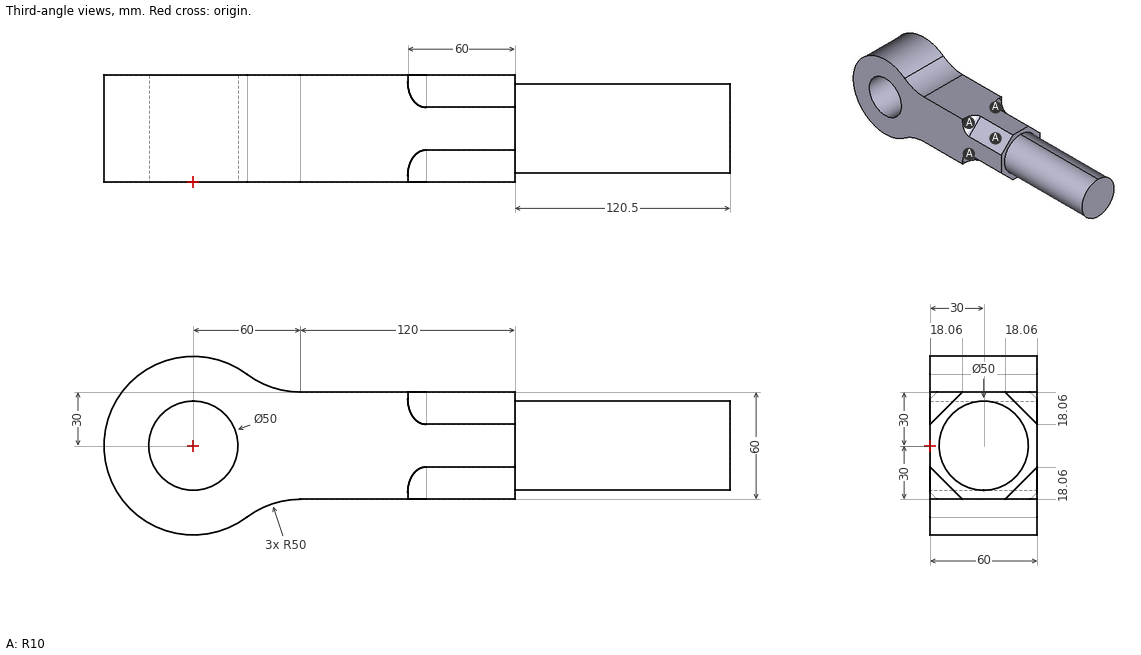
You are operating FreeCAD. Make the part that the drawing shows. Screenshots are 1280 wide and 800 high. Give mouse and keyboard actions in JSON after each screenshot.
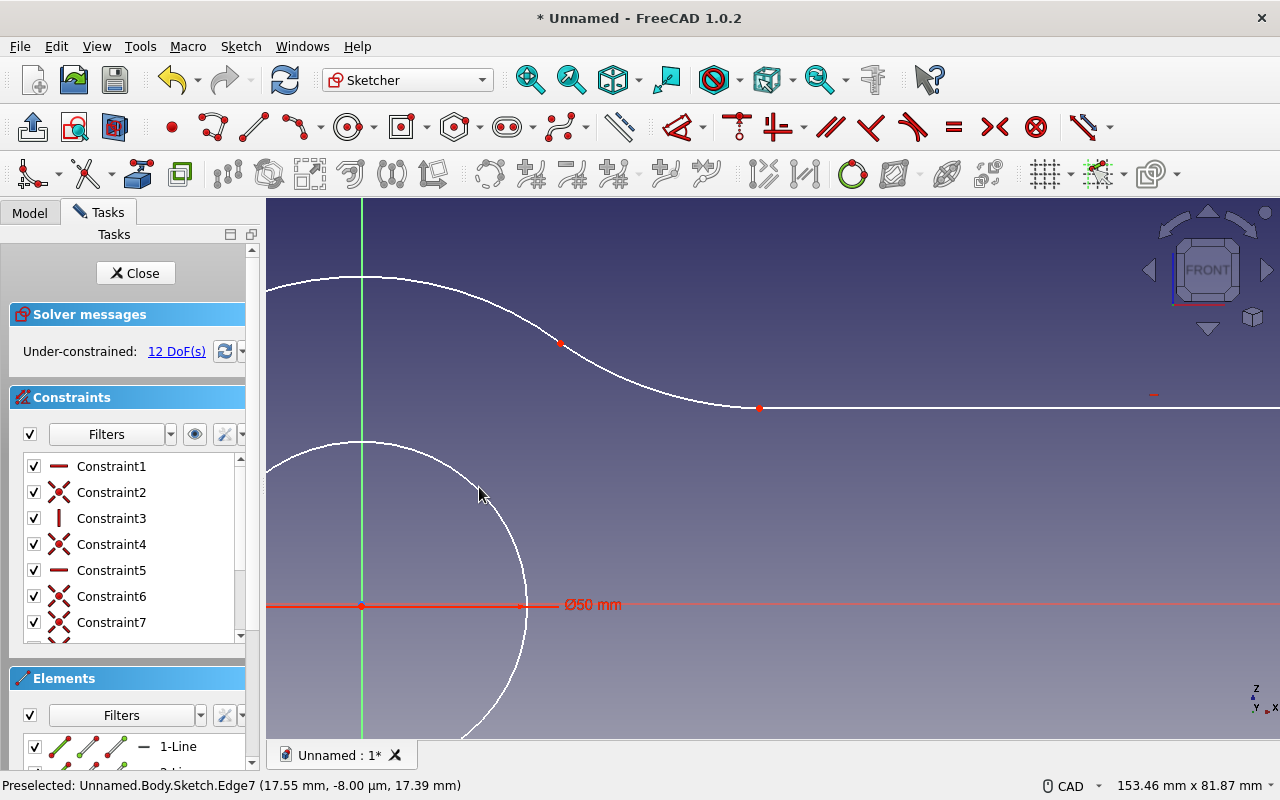
{"action": "scroll", "coordinate": [654, 389], "scroll_direction": "down", "scroll_amount": 5}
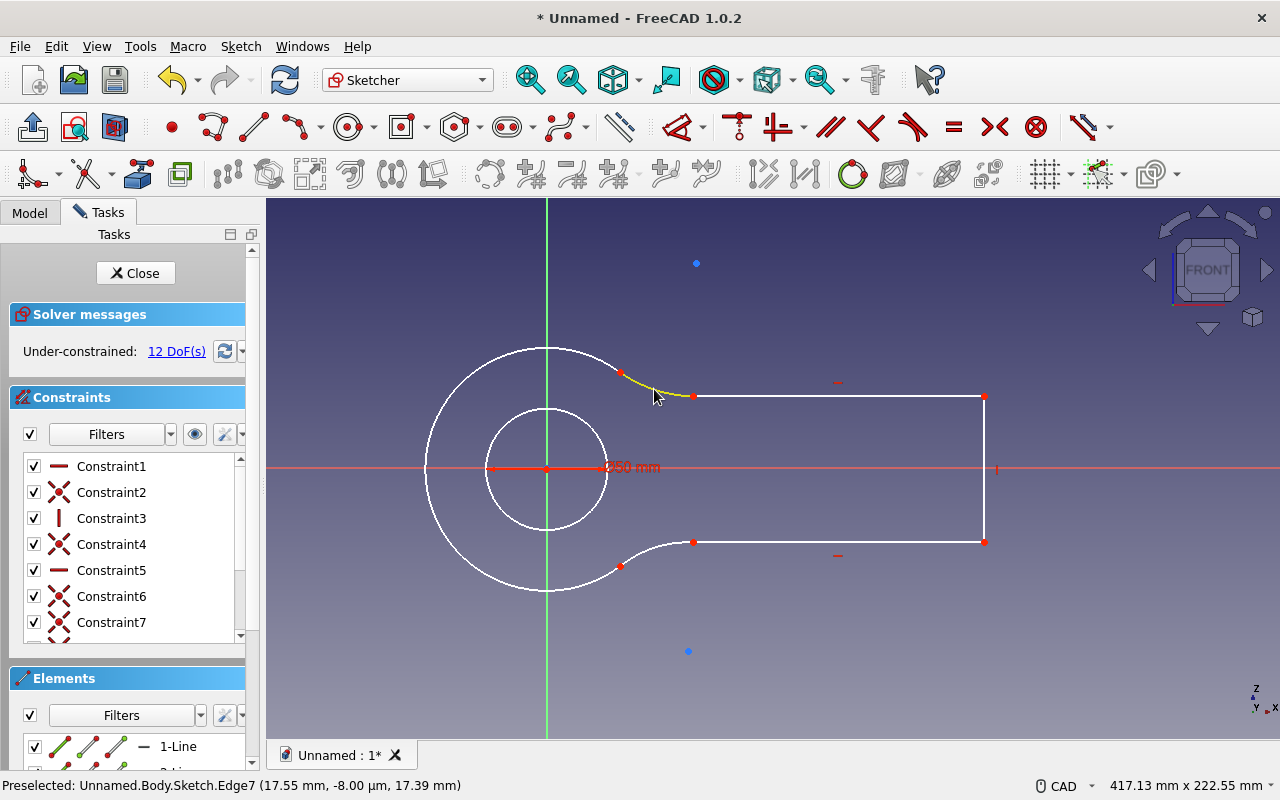
{"action": "left_click", "coordinate": [670, 544]}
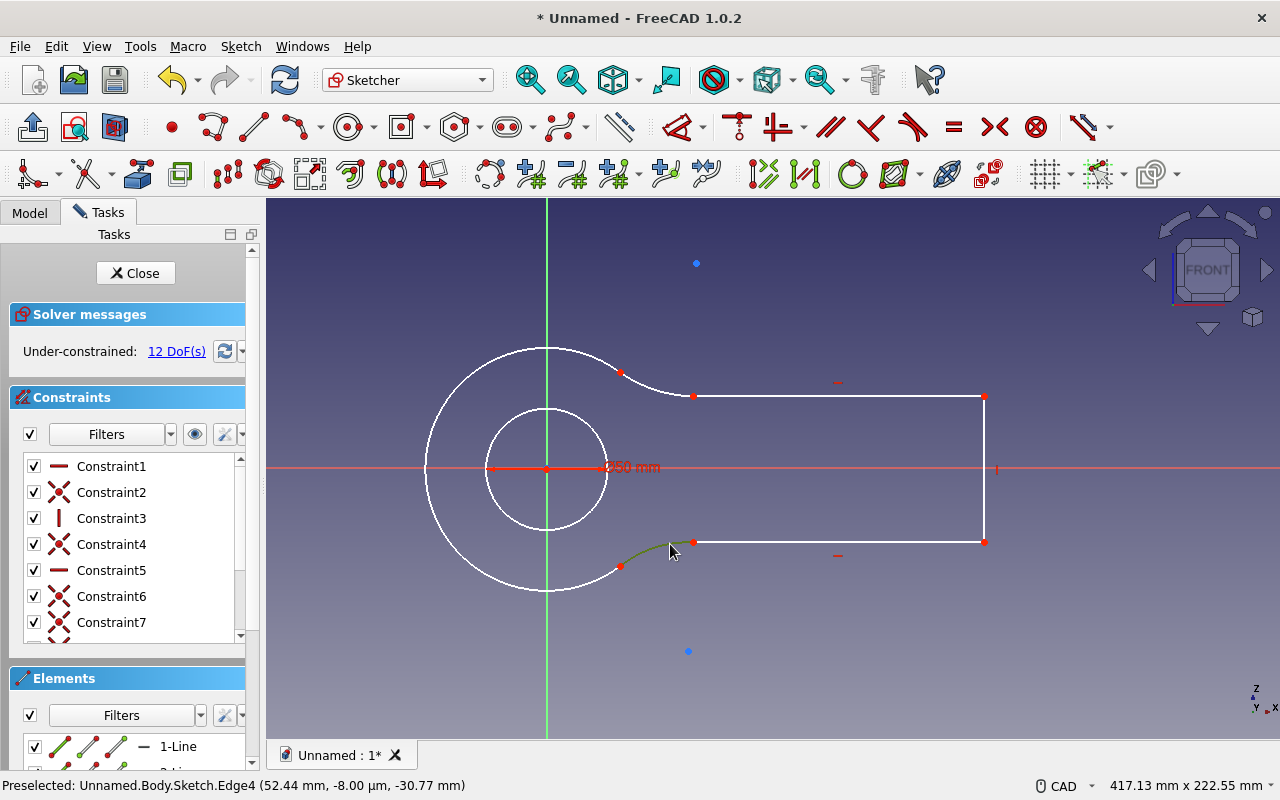
{"action": "left_click", "coordinate": [470, 375]}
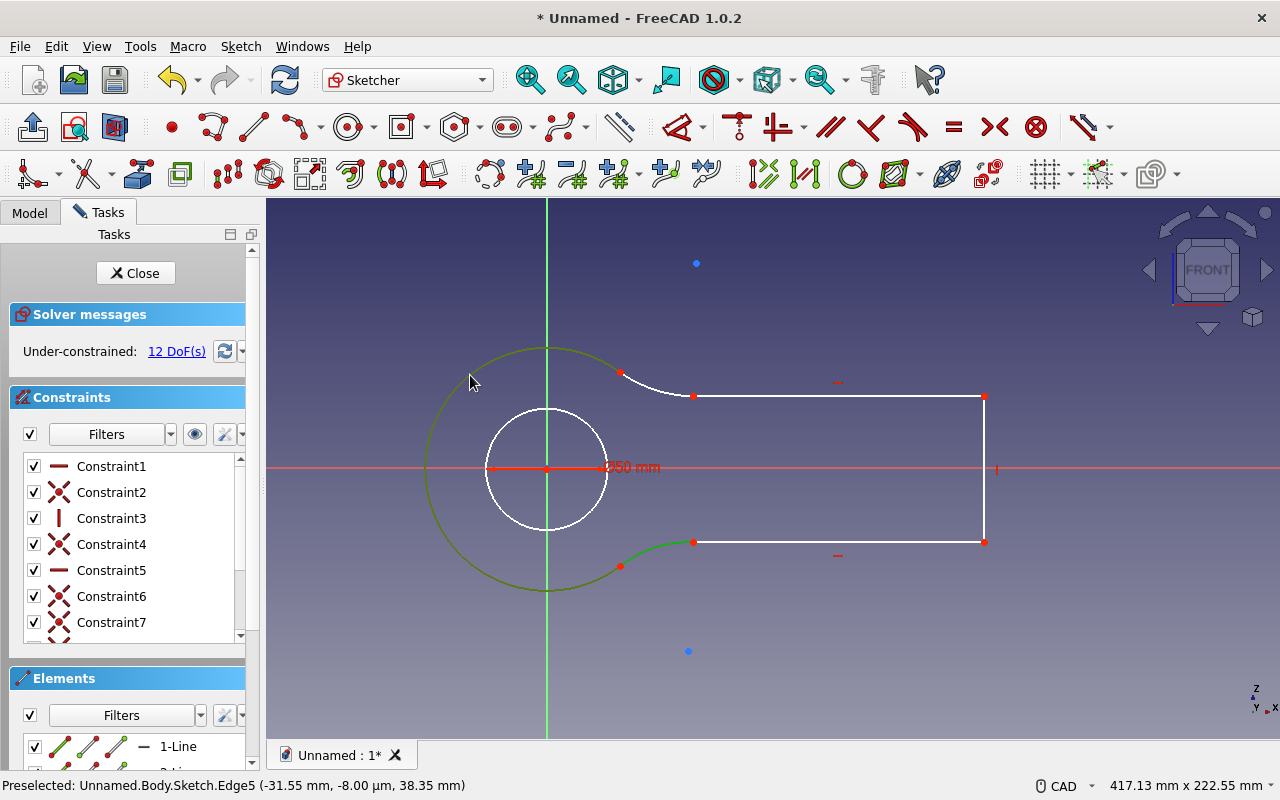
{"action": "key", "text": "t"}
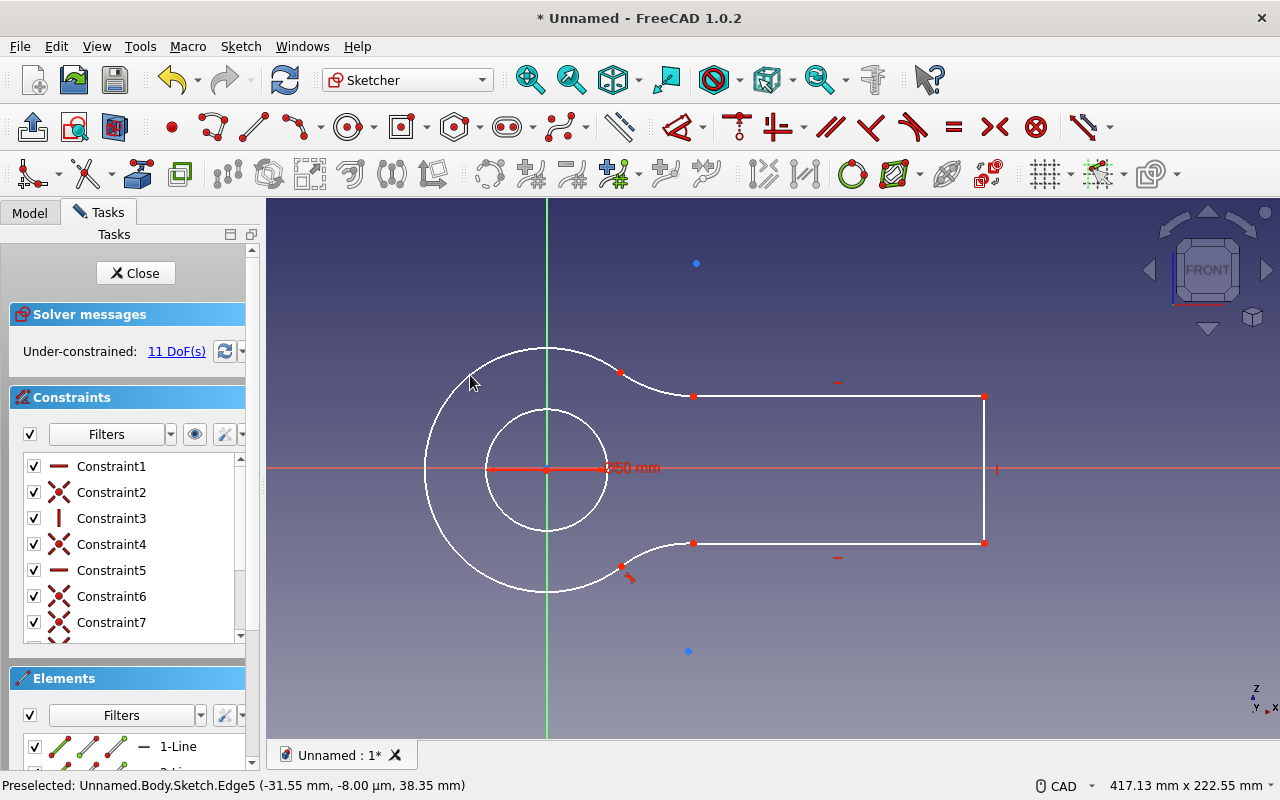
{"action": "left_click", "coordinate": [469, 376]}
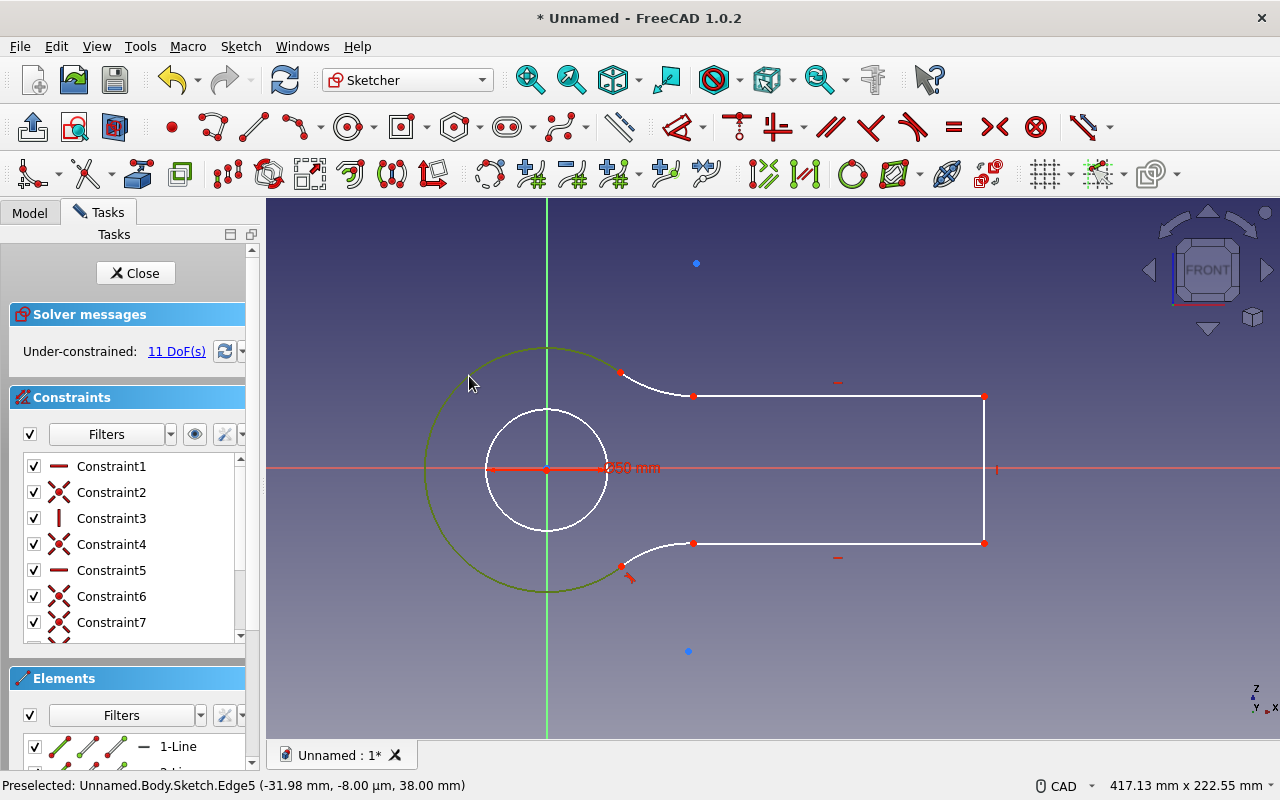
{"action": "left_click", "coordinate": [640, 384]}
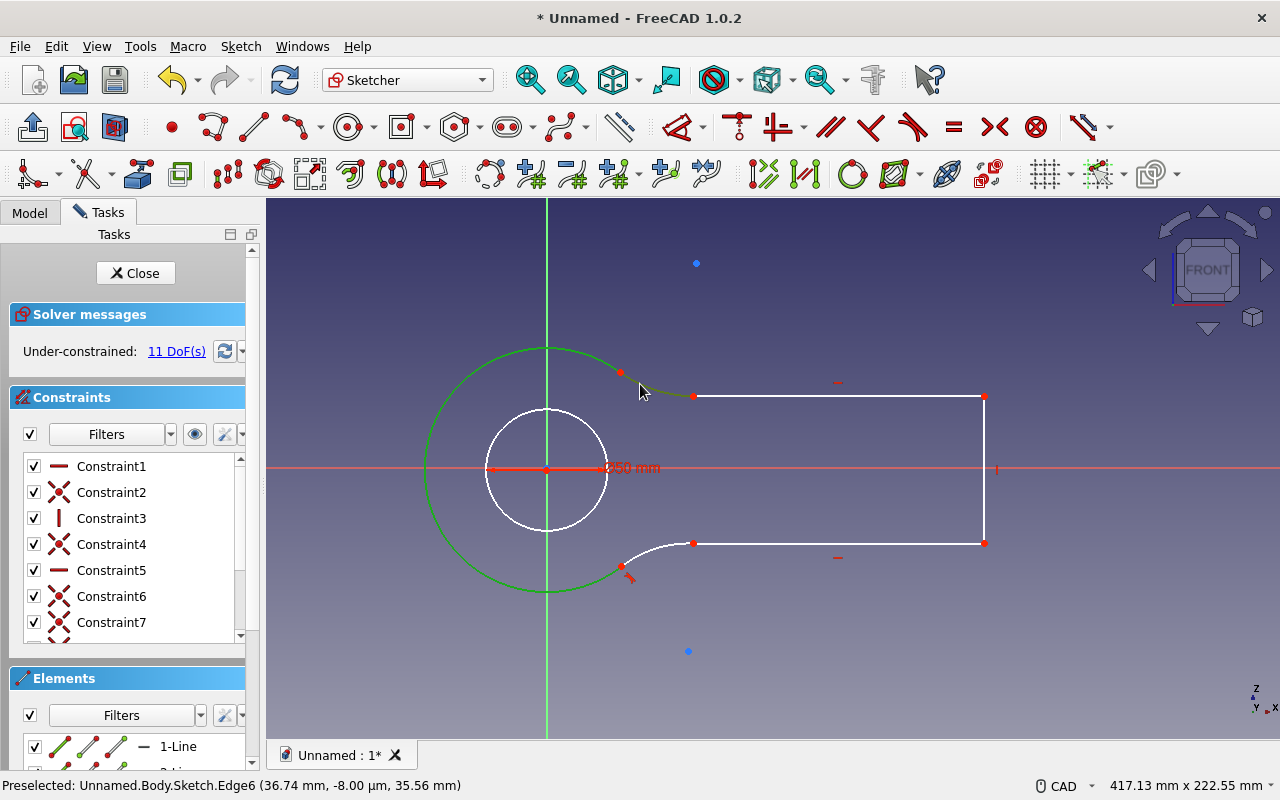
{"action": "key", "text": "t"}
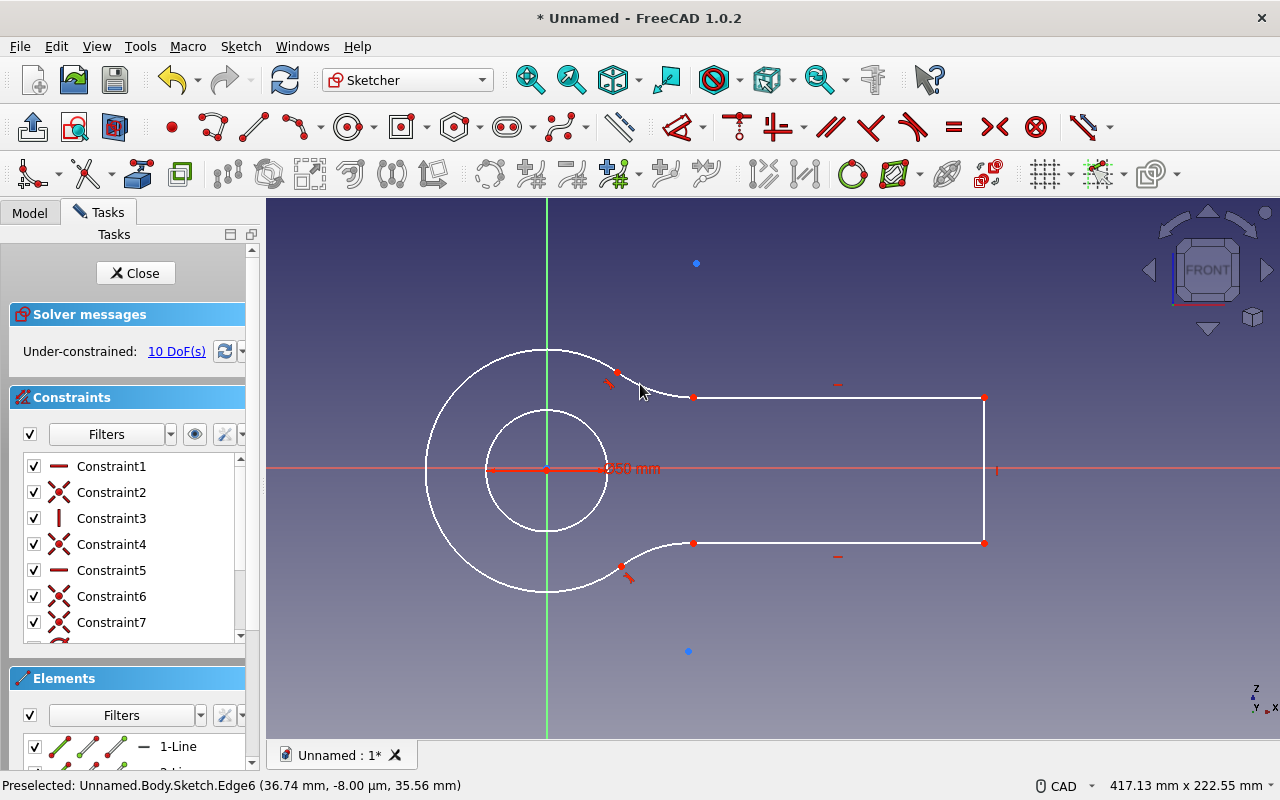
{"action": "left_click_drag", "start_coordinate": [537, 458], "coordinate": [557, 481]}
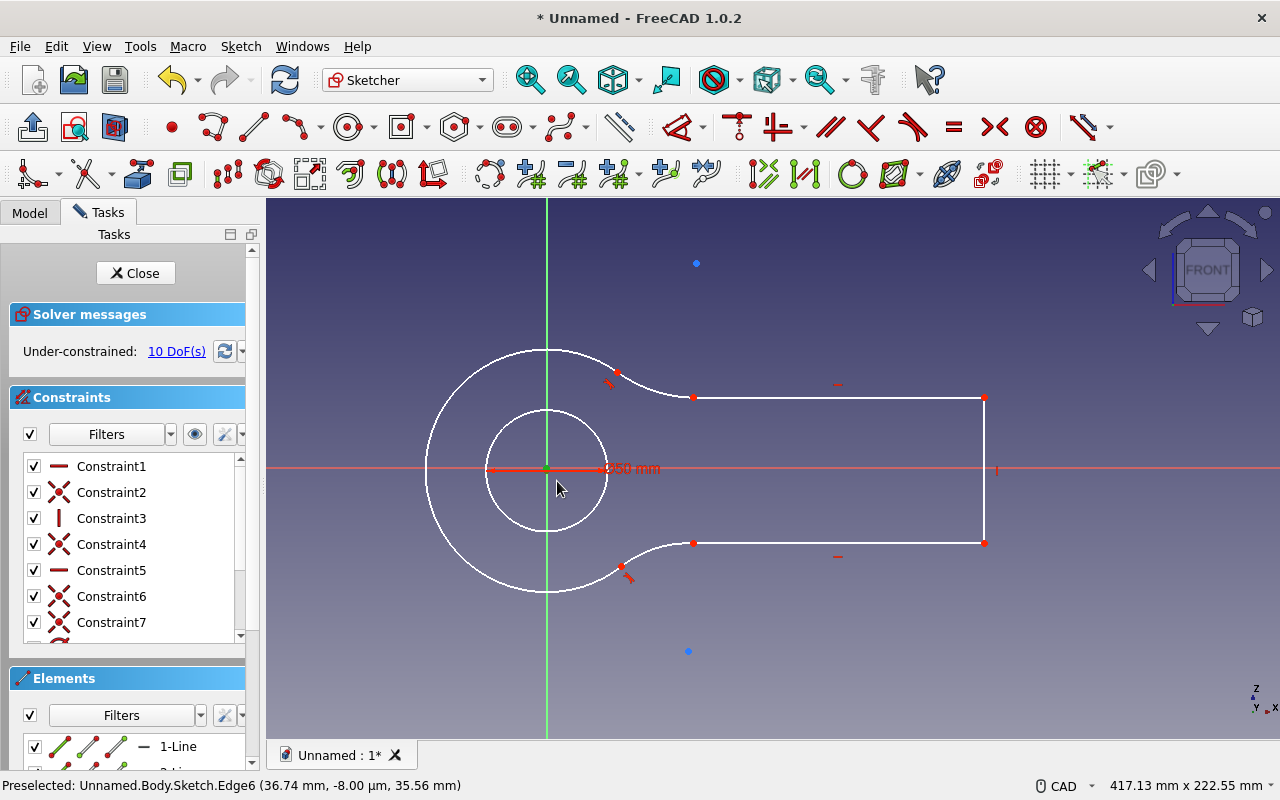
{"action": "key", "text": "c"}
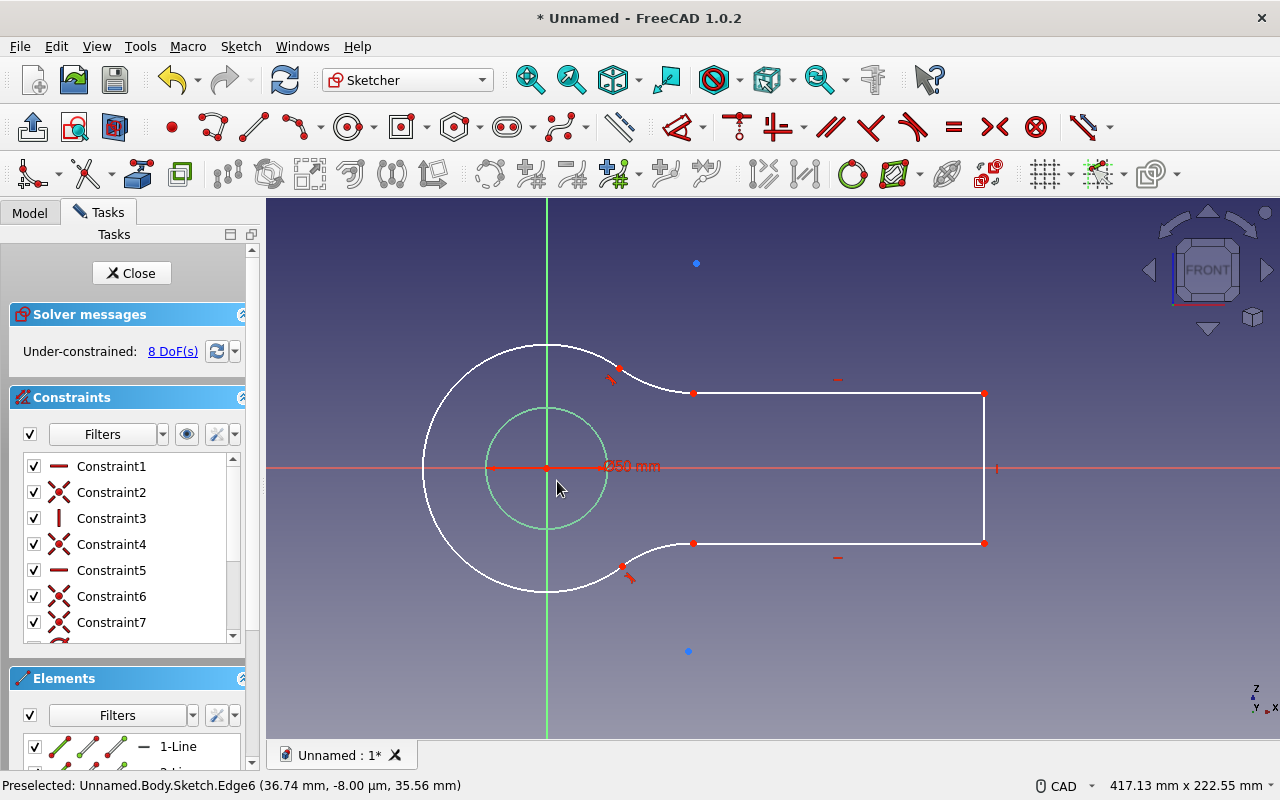
{"action": "left_click", "coordinate": [670, 545]}